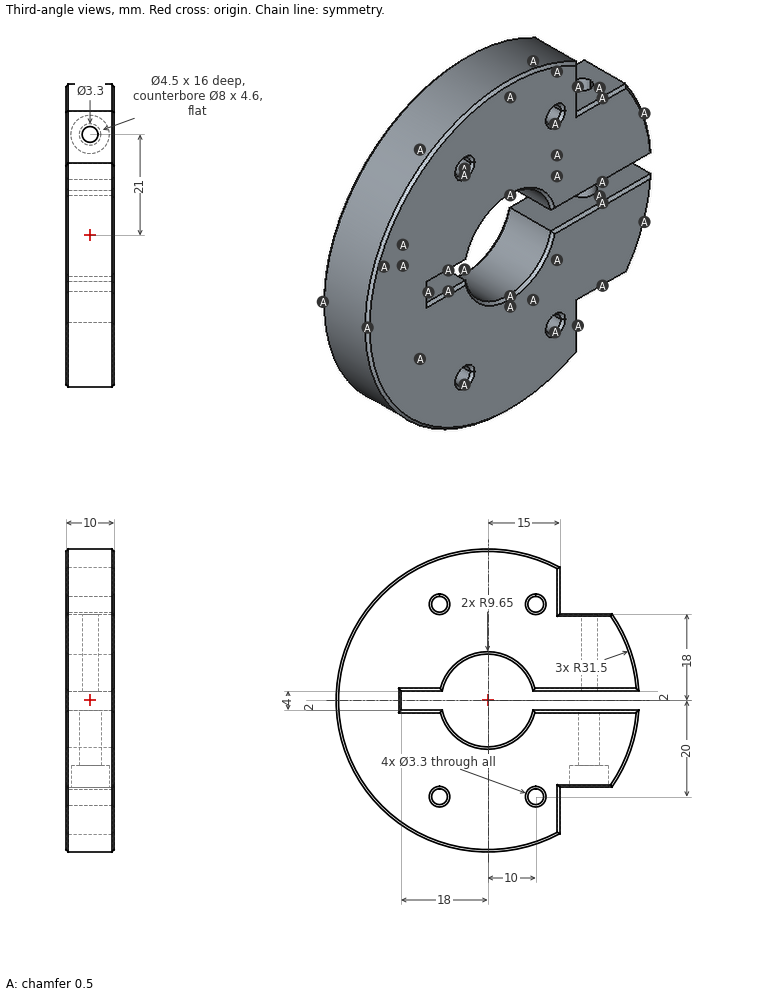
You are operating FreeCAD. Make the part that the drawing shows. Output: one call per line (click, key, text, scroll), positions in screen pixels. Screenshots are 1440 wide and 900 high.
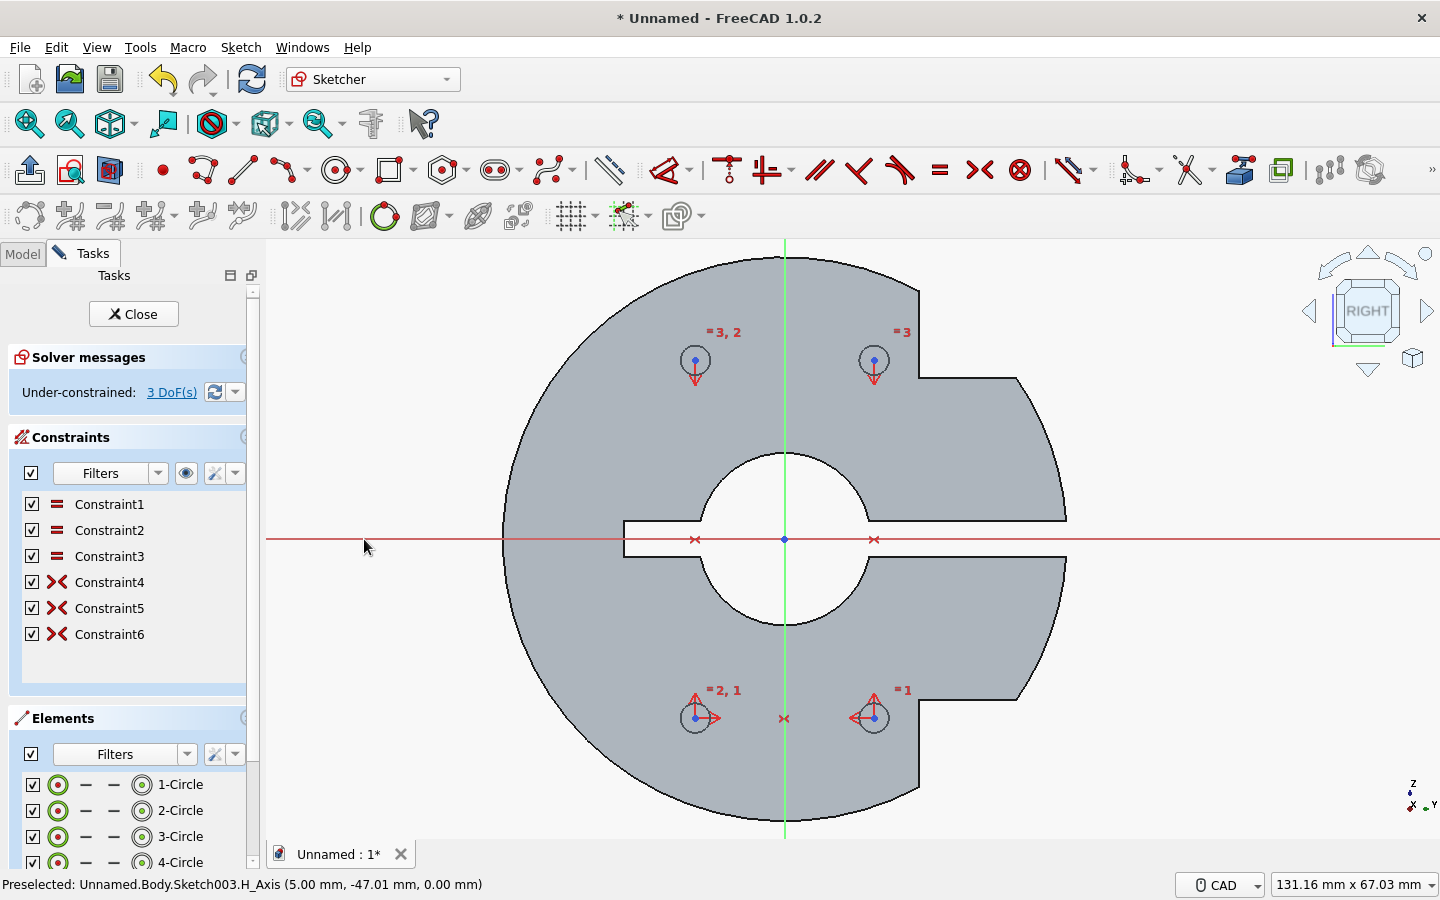
scroll(885, 708, up, 2)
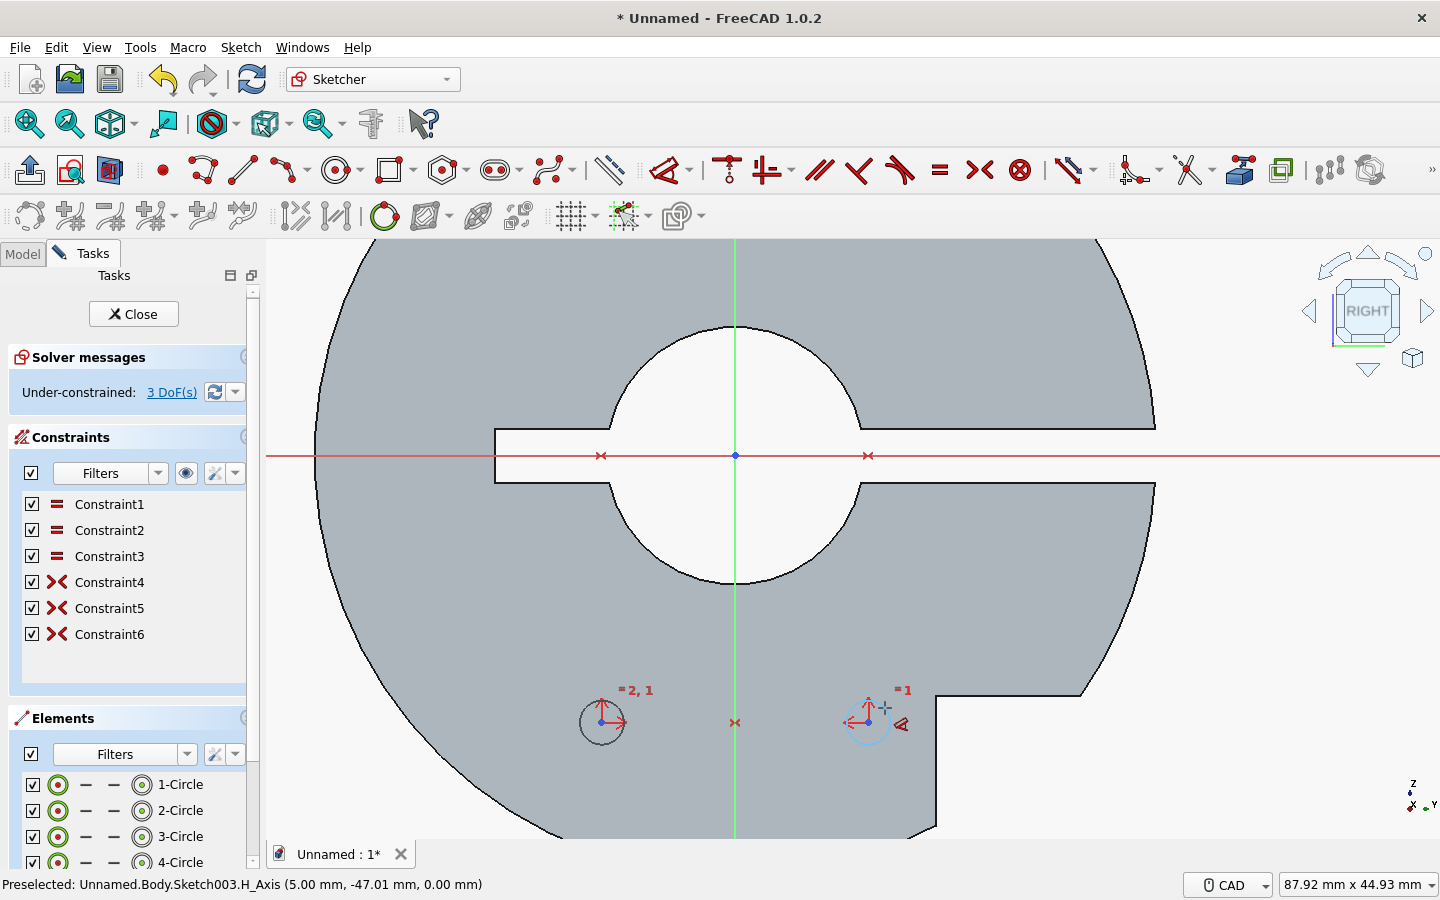
click(884, 707)
click(906, 684)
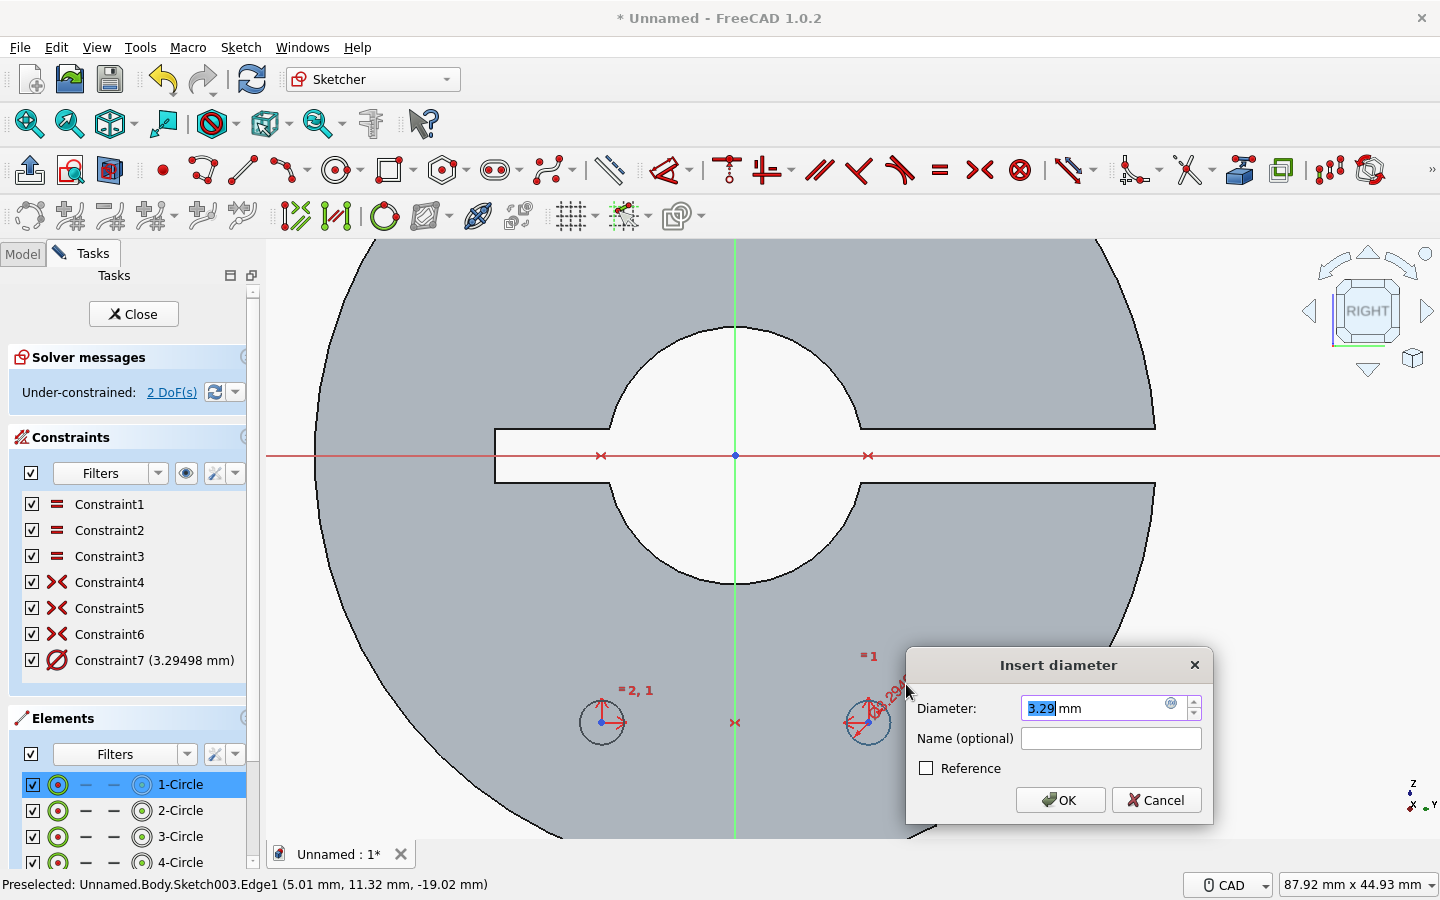
text(3.3)
key(Return)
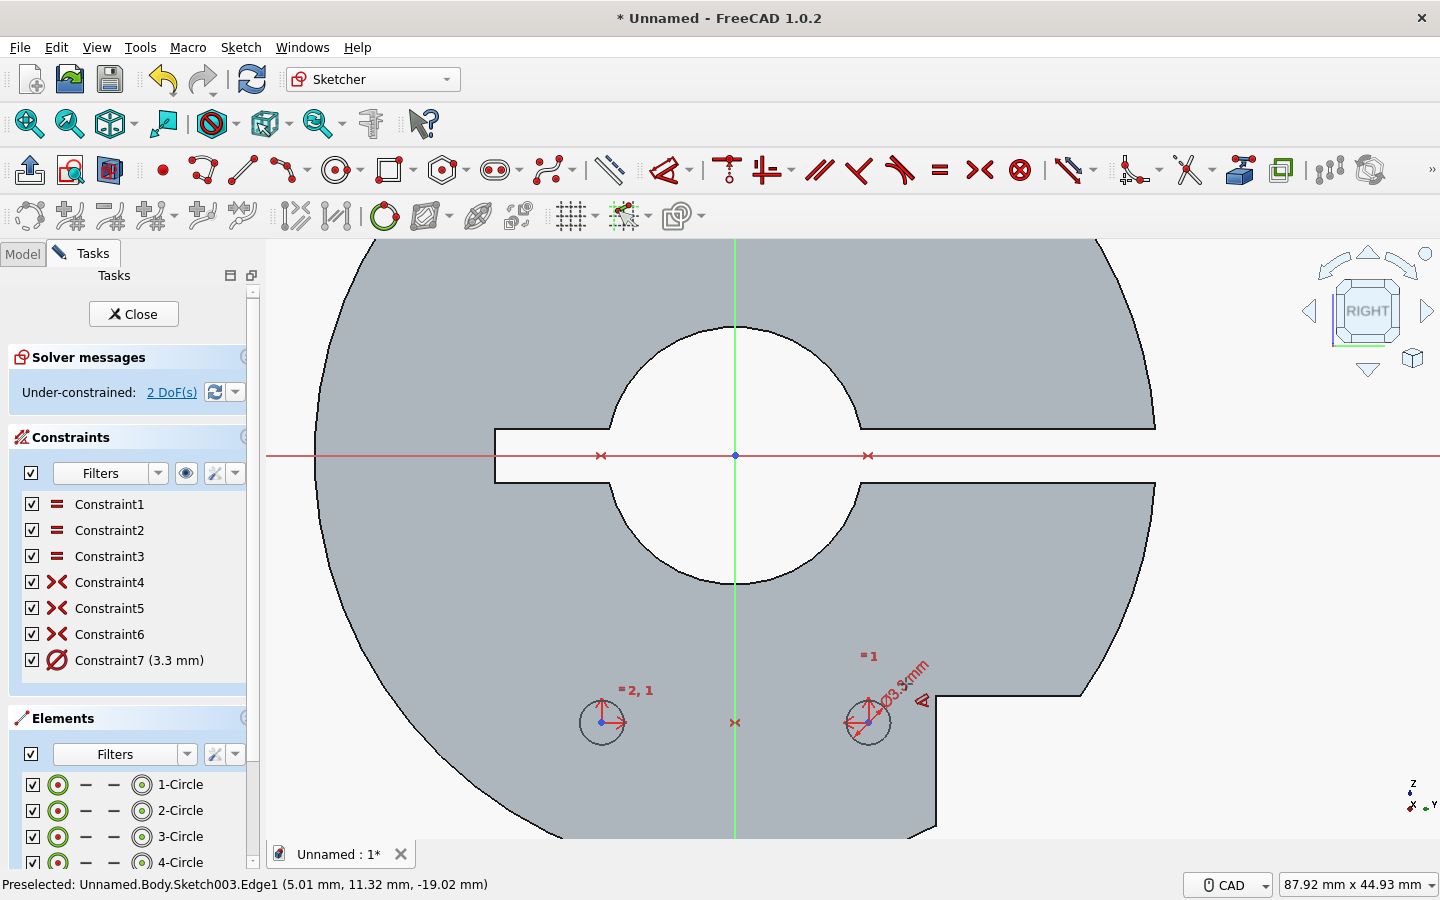
click(869, 723)
click(802, 757)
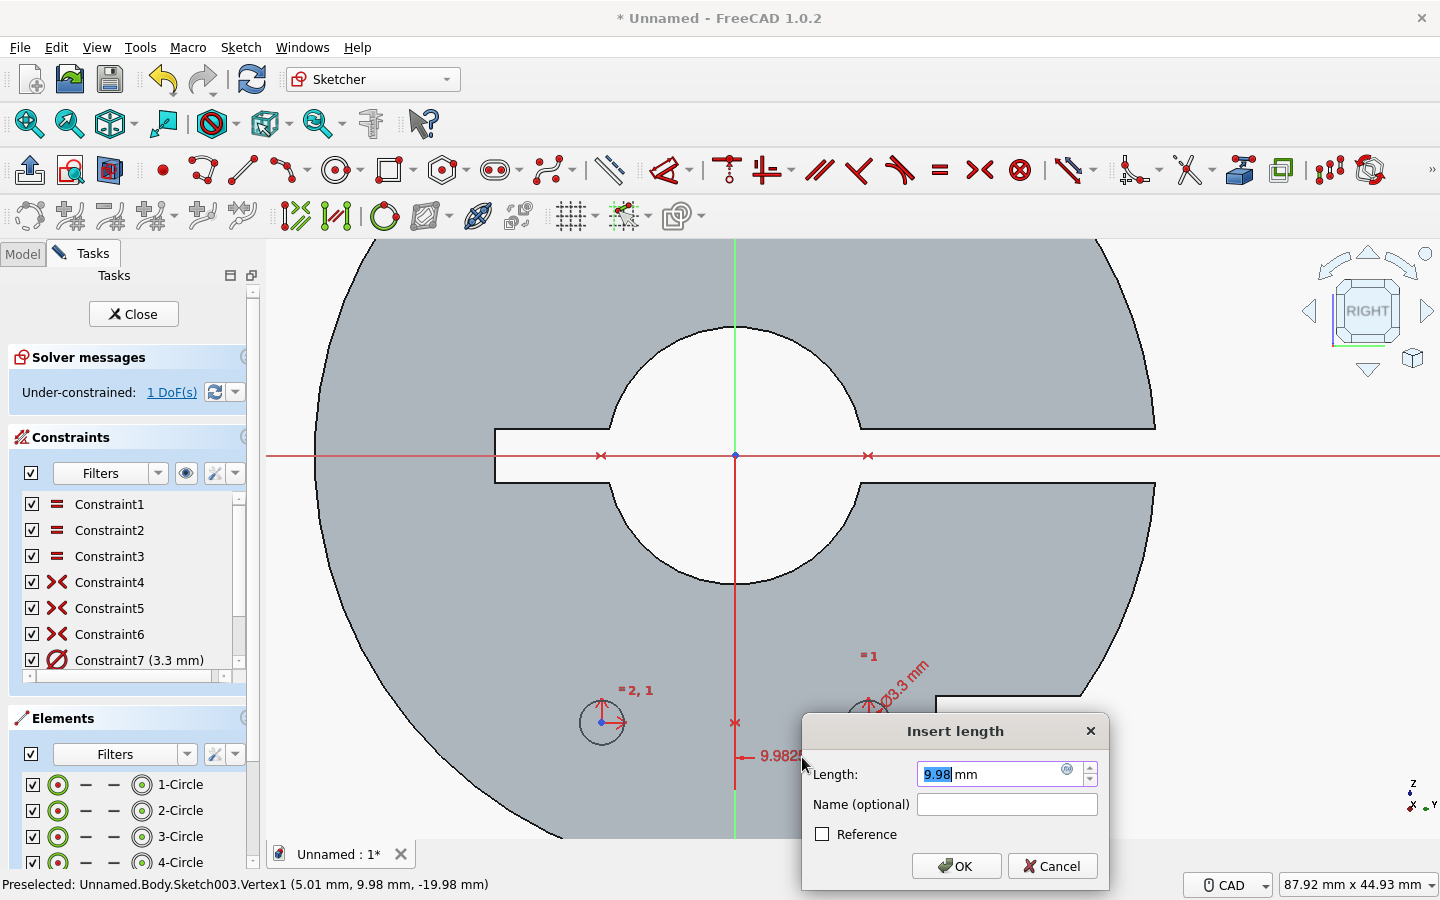
text(10)
key(Return)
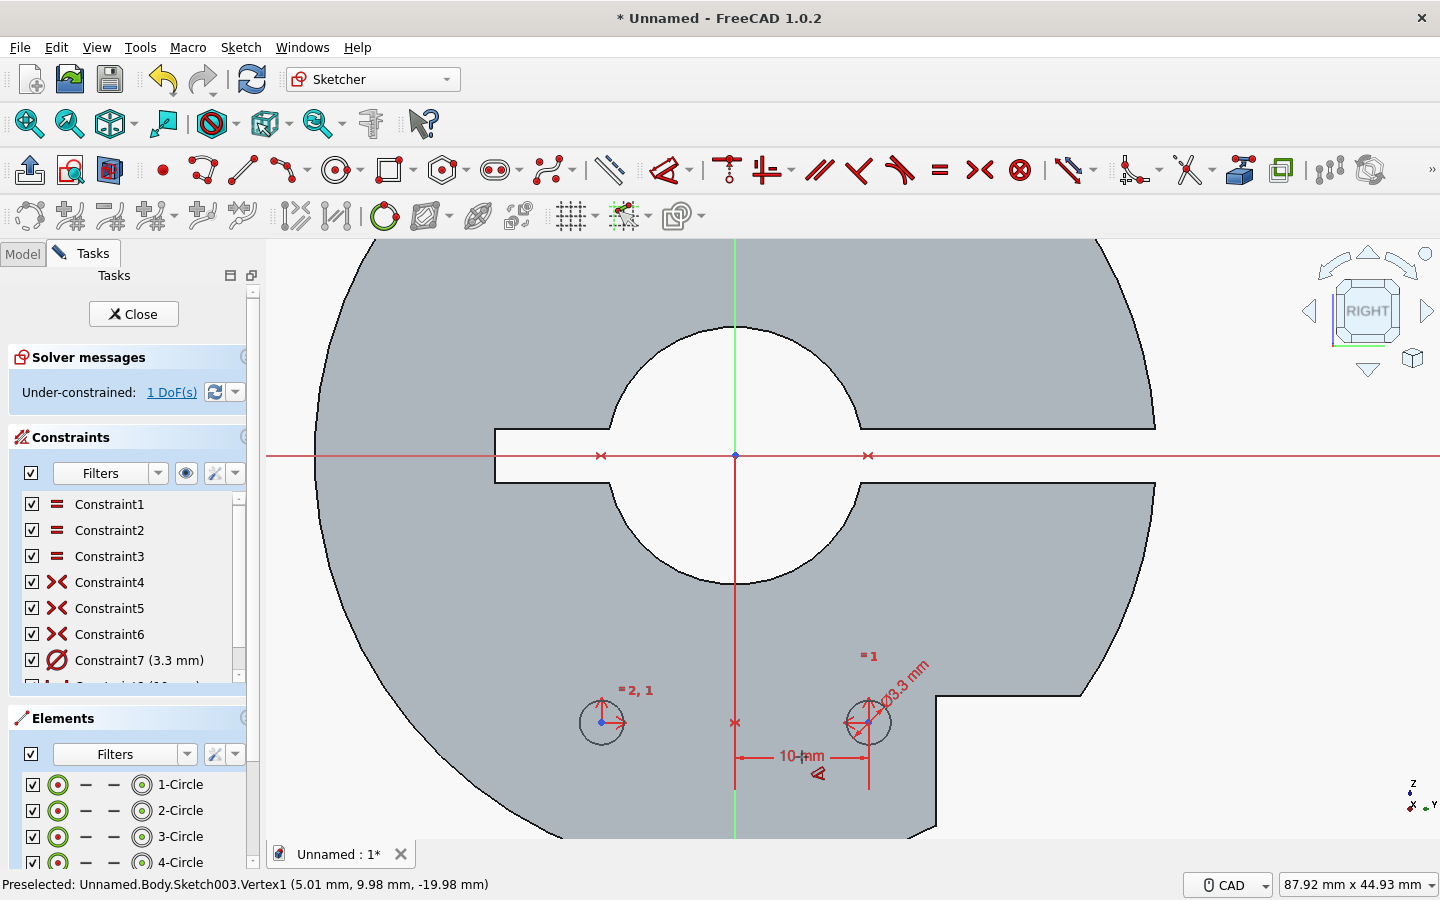
click(869, 723)
click(903, 589)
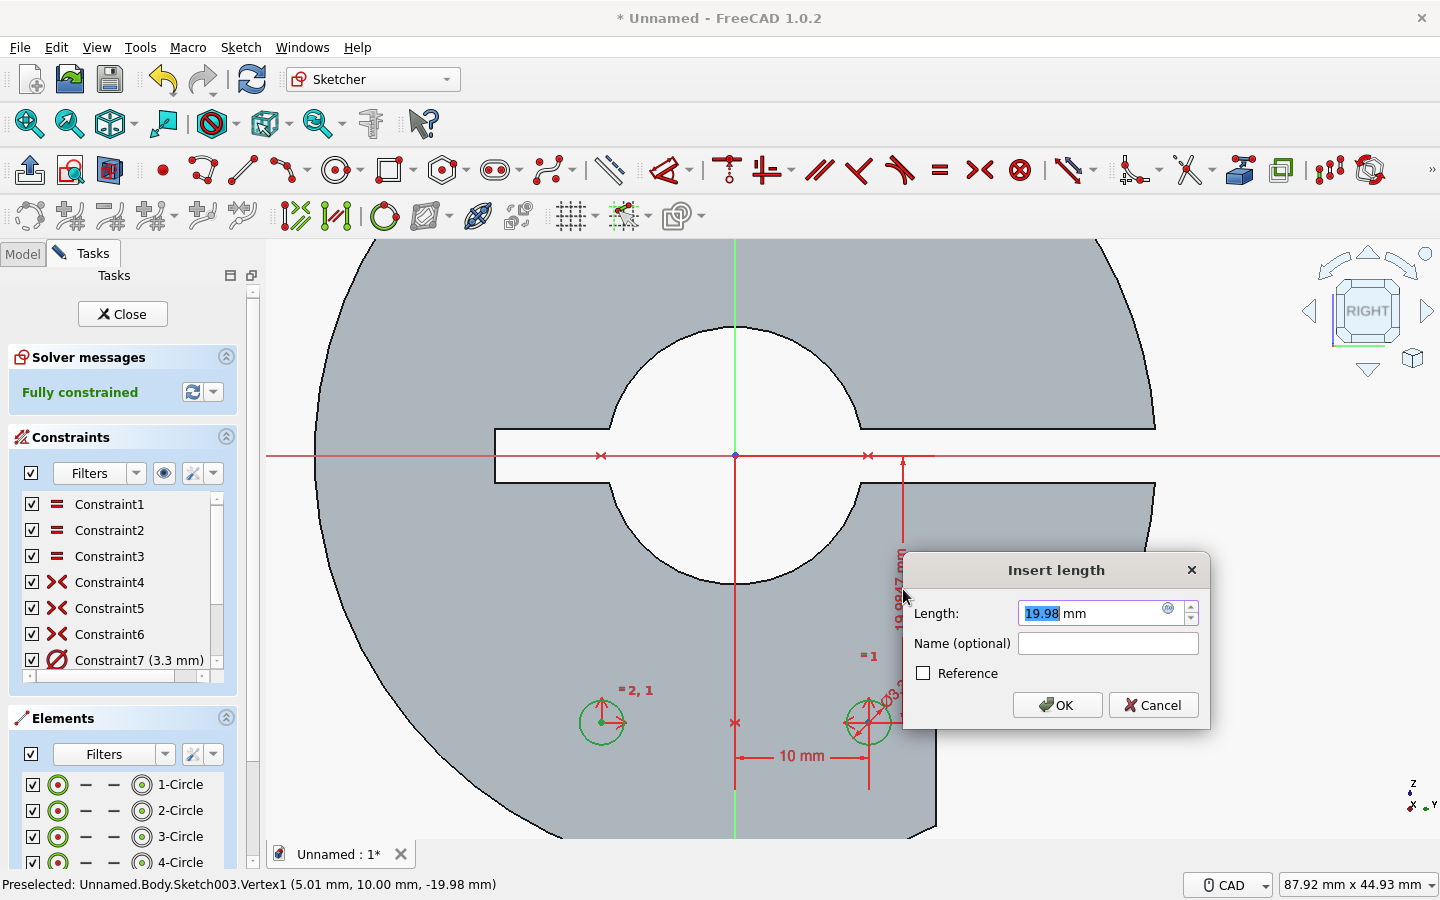
text(20)
key(Return)
key(Escape)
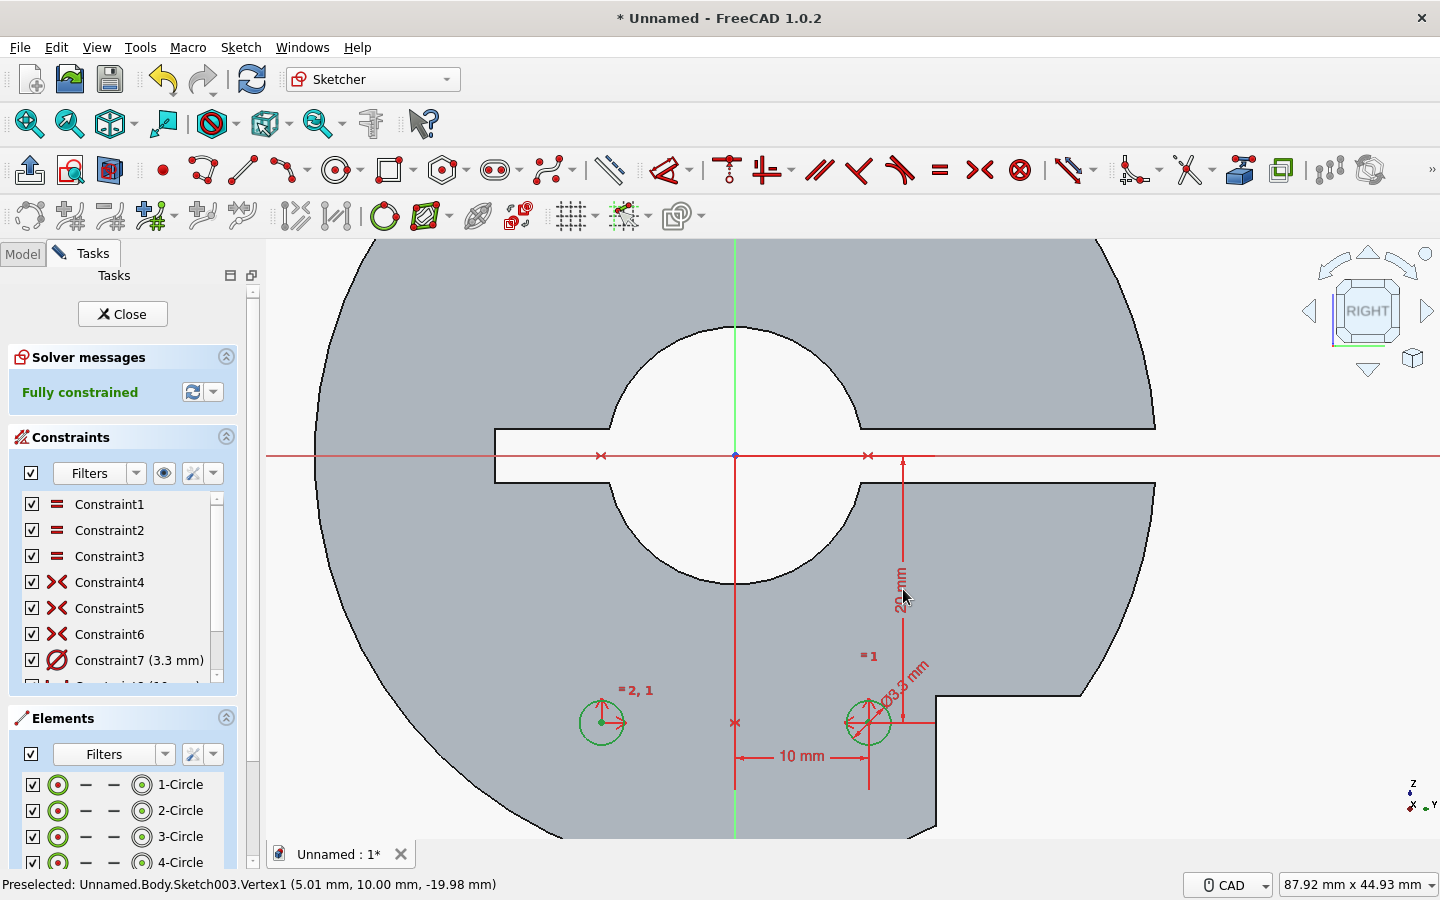
click(123, 314)